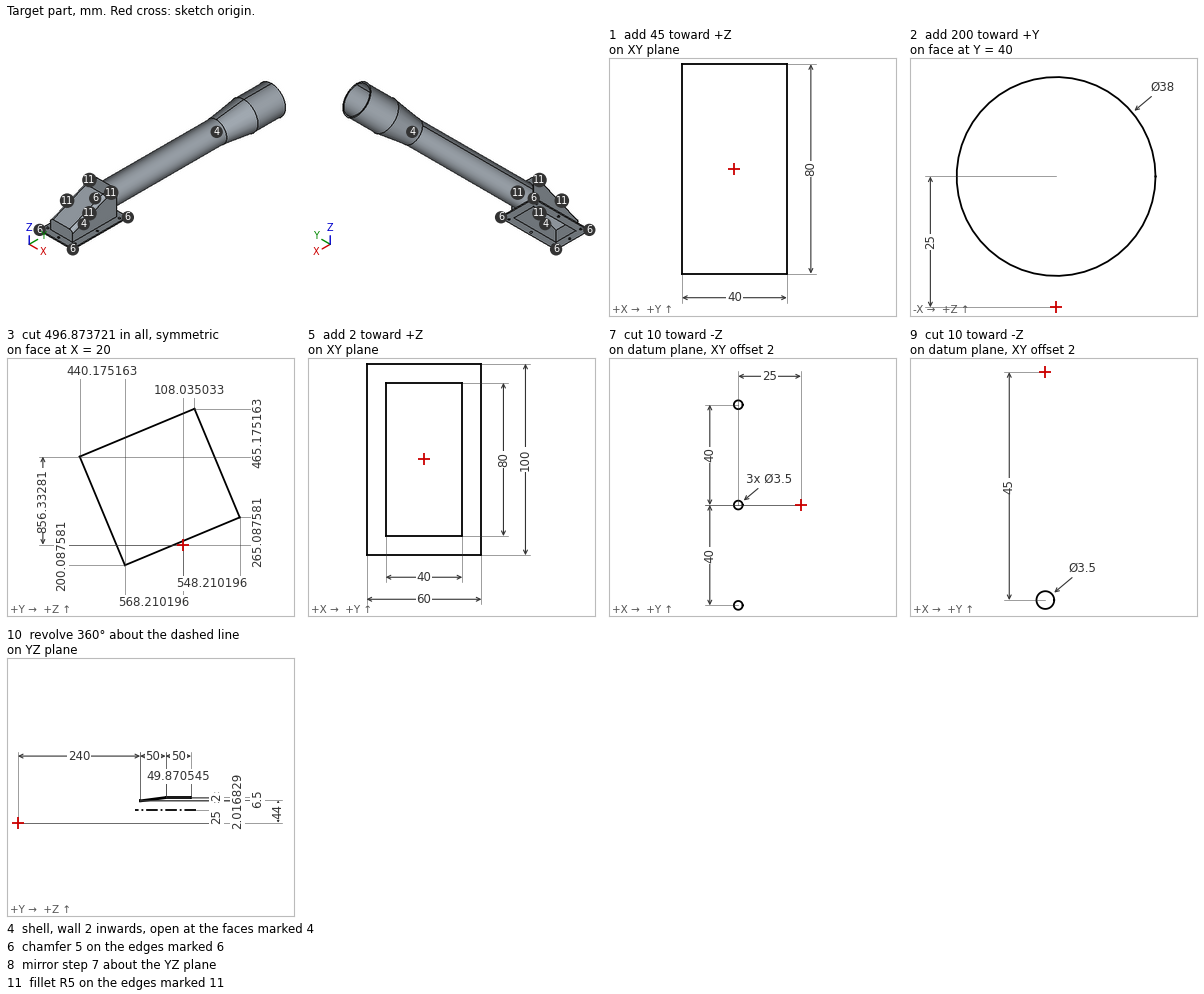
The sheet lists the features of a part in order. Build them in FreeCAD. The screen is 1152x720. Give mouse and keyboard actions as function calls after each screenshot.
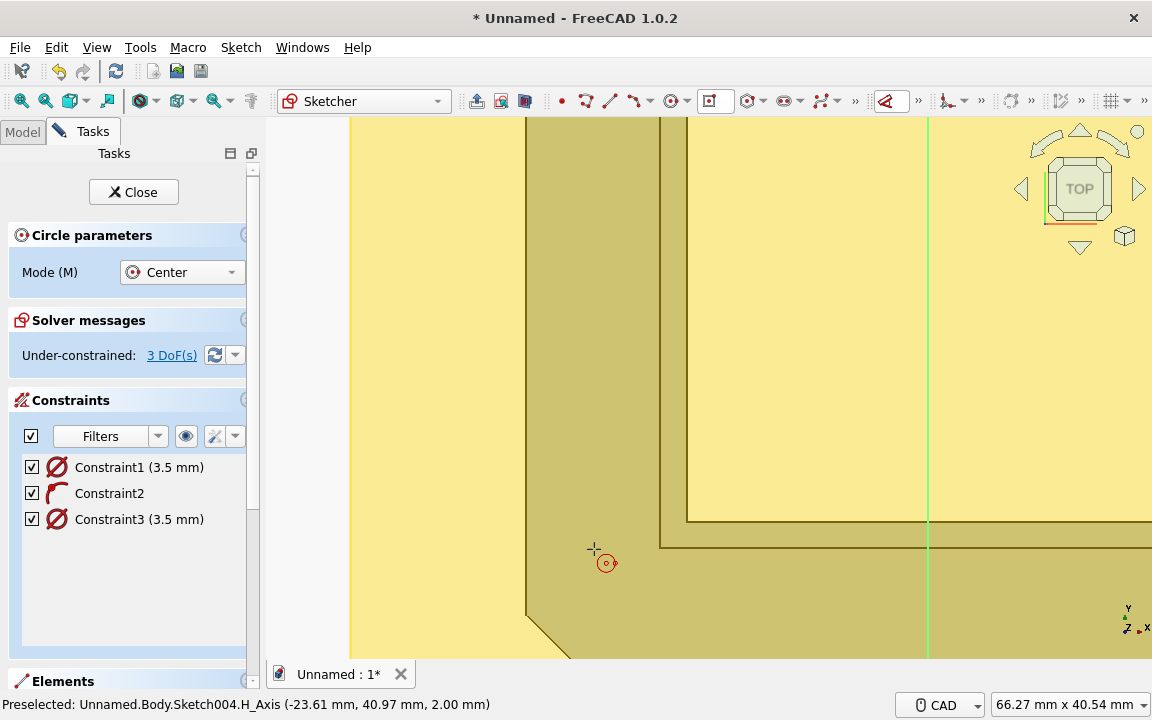
click(593, 548)
move(610, 532)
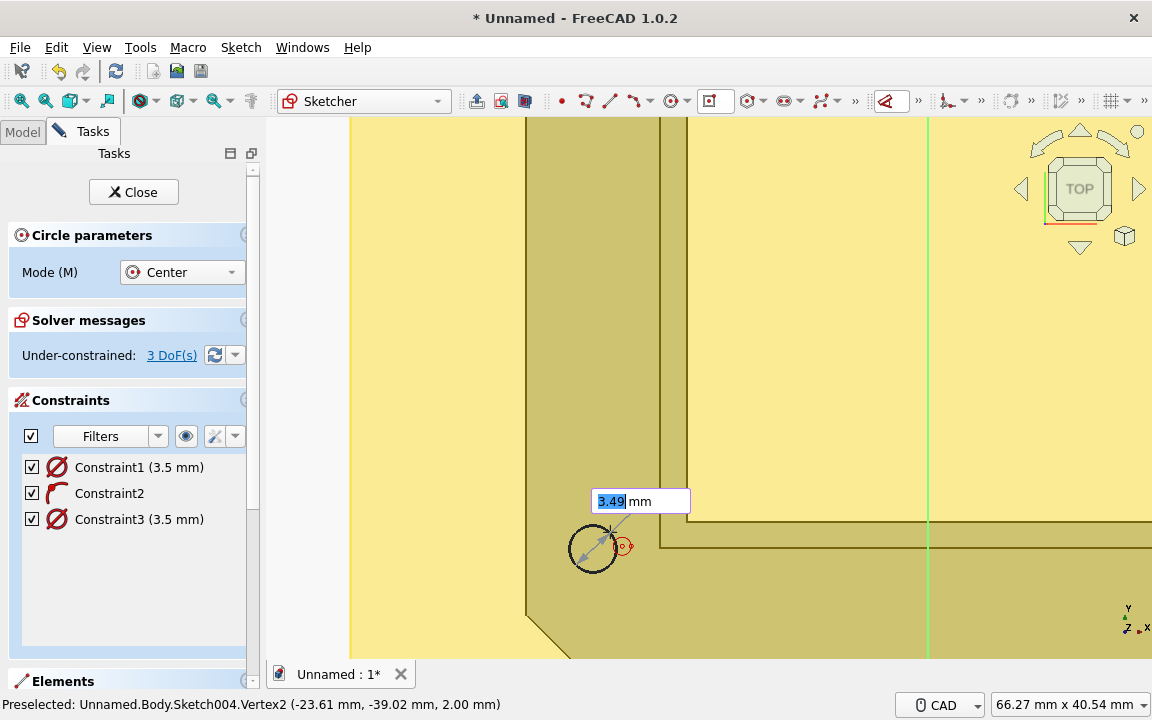
text(3.5)
key(Return)
key(Escape)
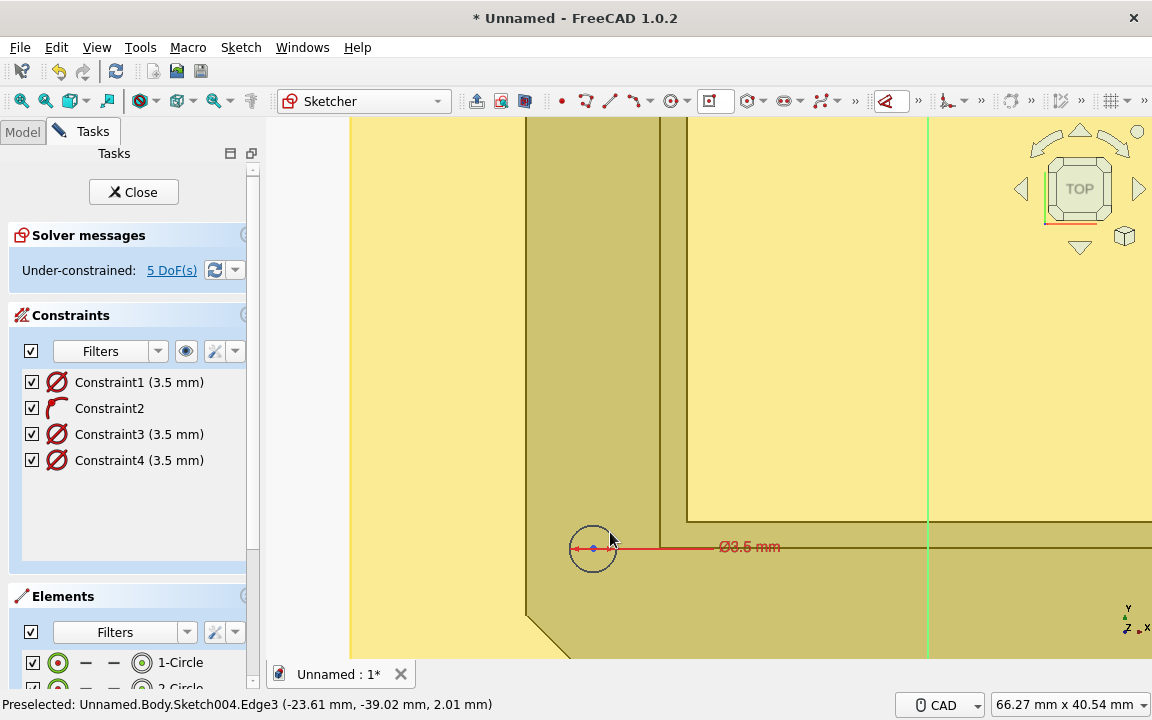
scroll(594, 549, down, 6)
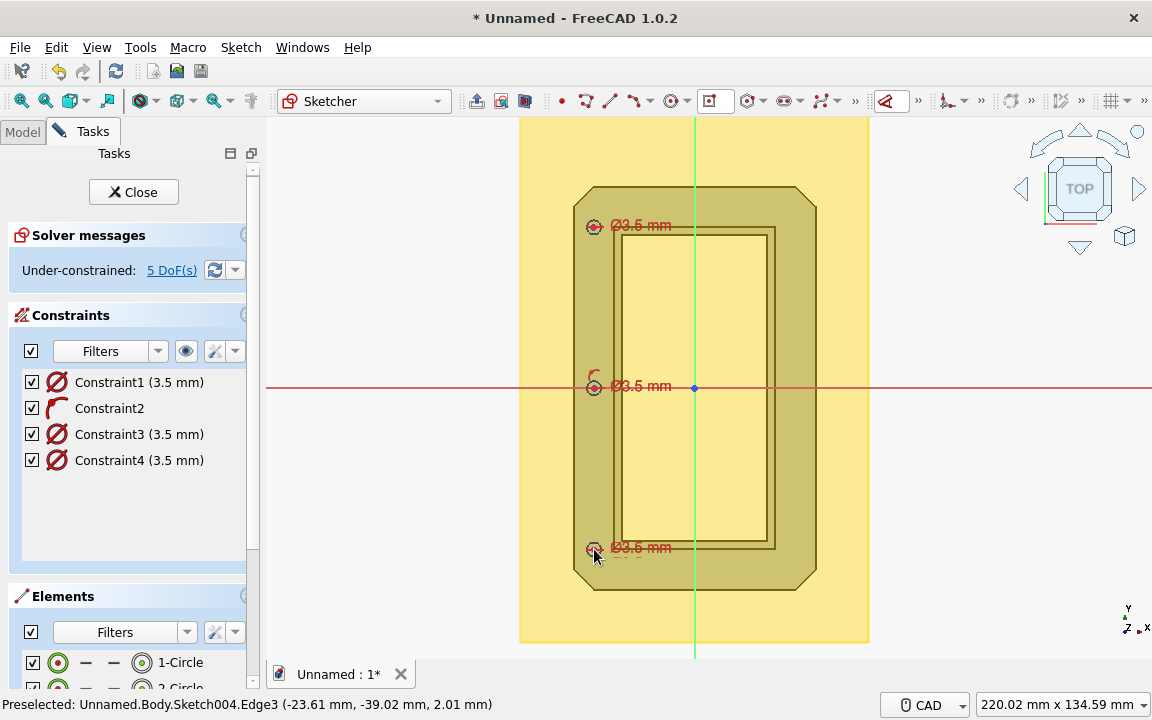
click(594, 388)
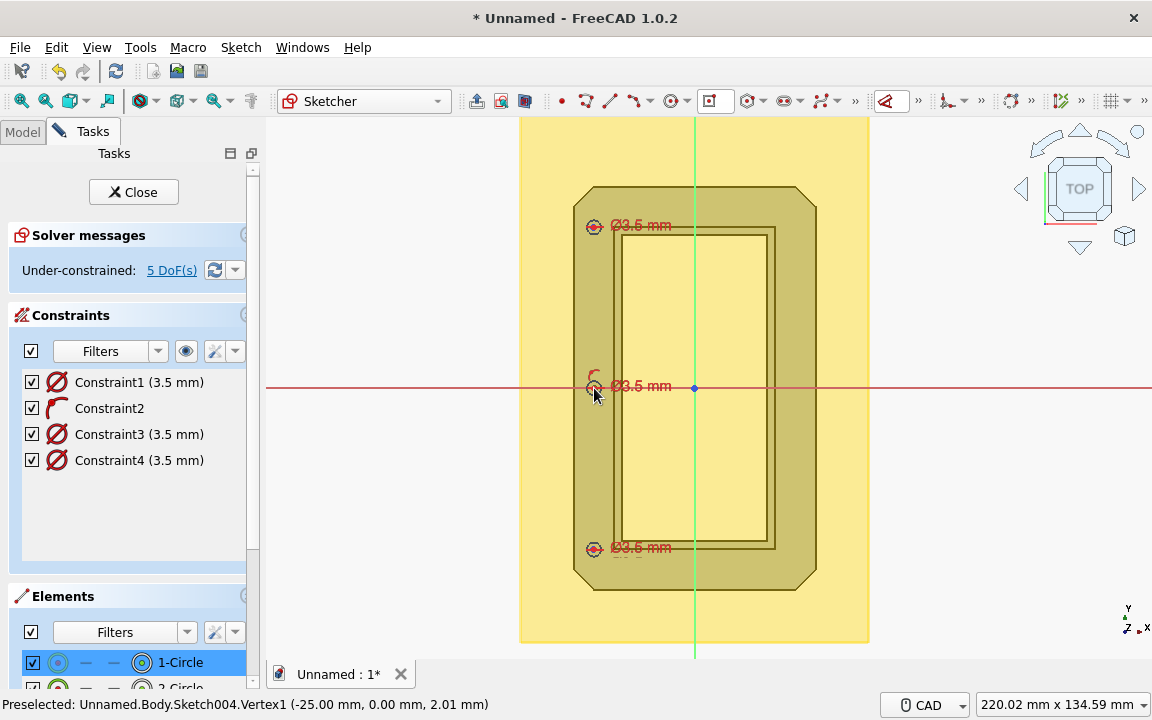
click(594, 227)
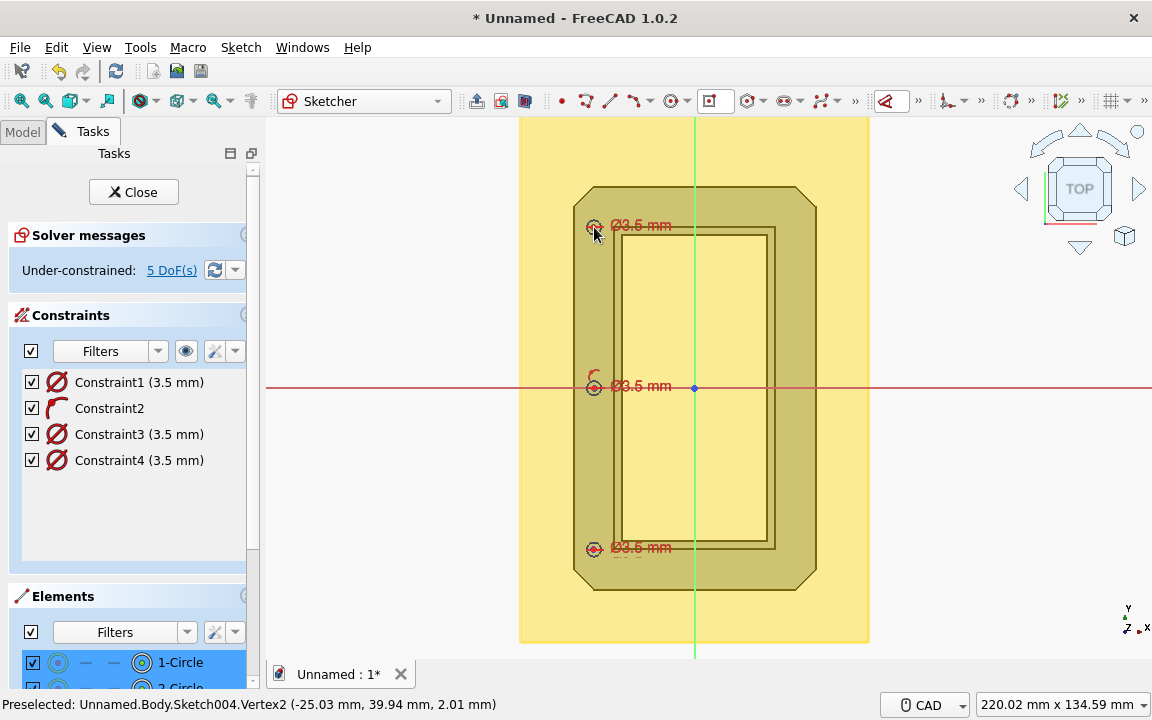
key(v)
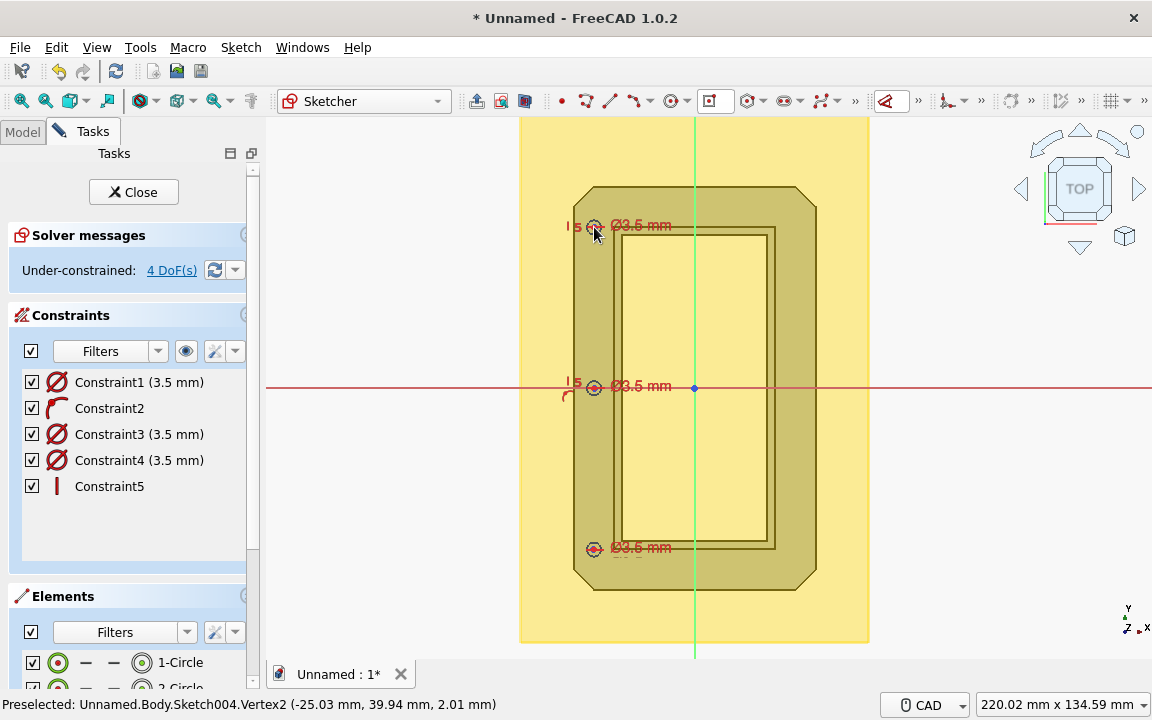
click(594, 388)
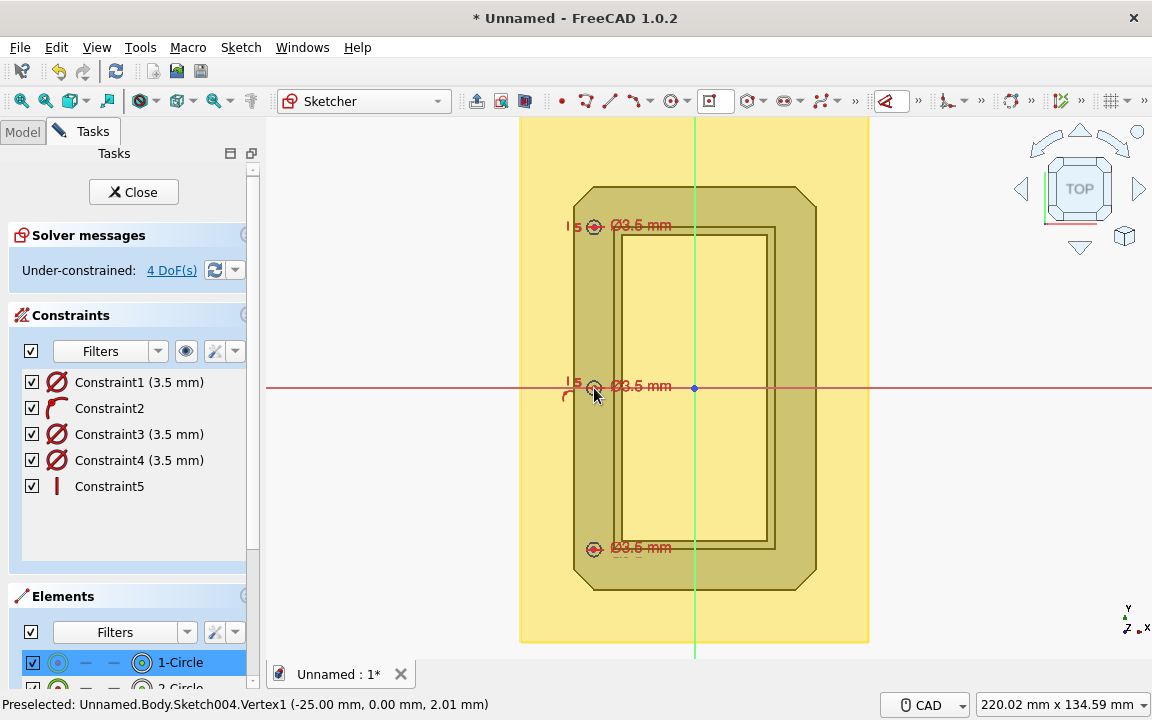
click(594, 550)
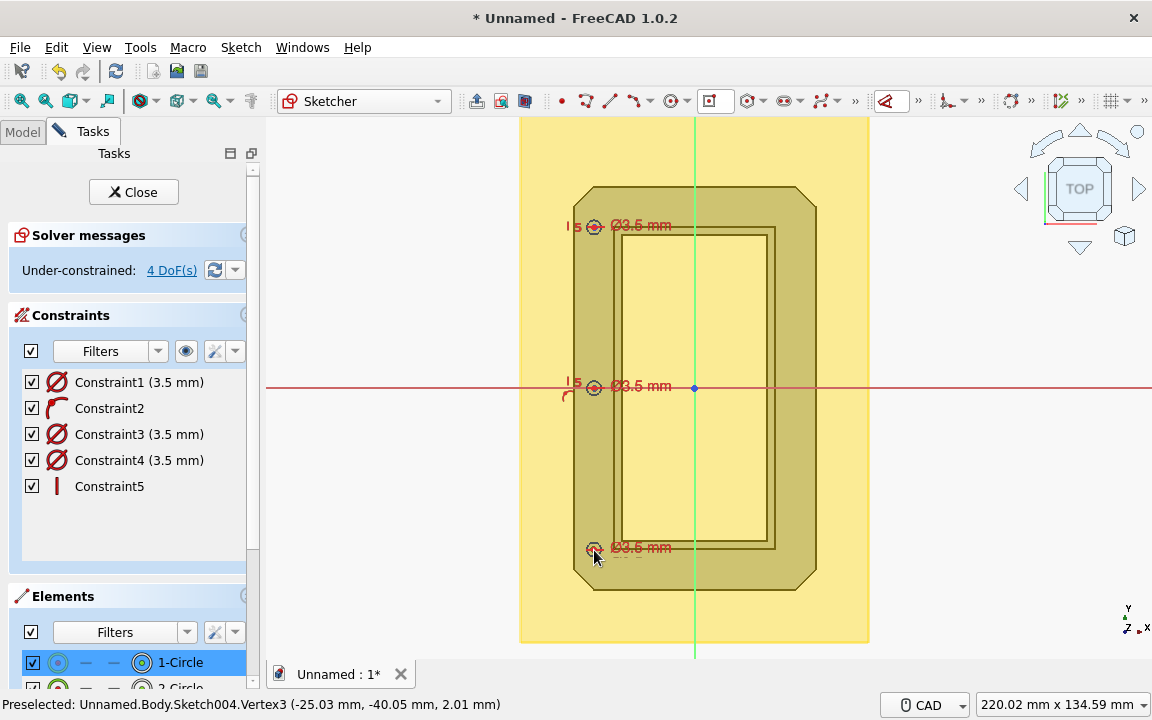
key(v)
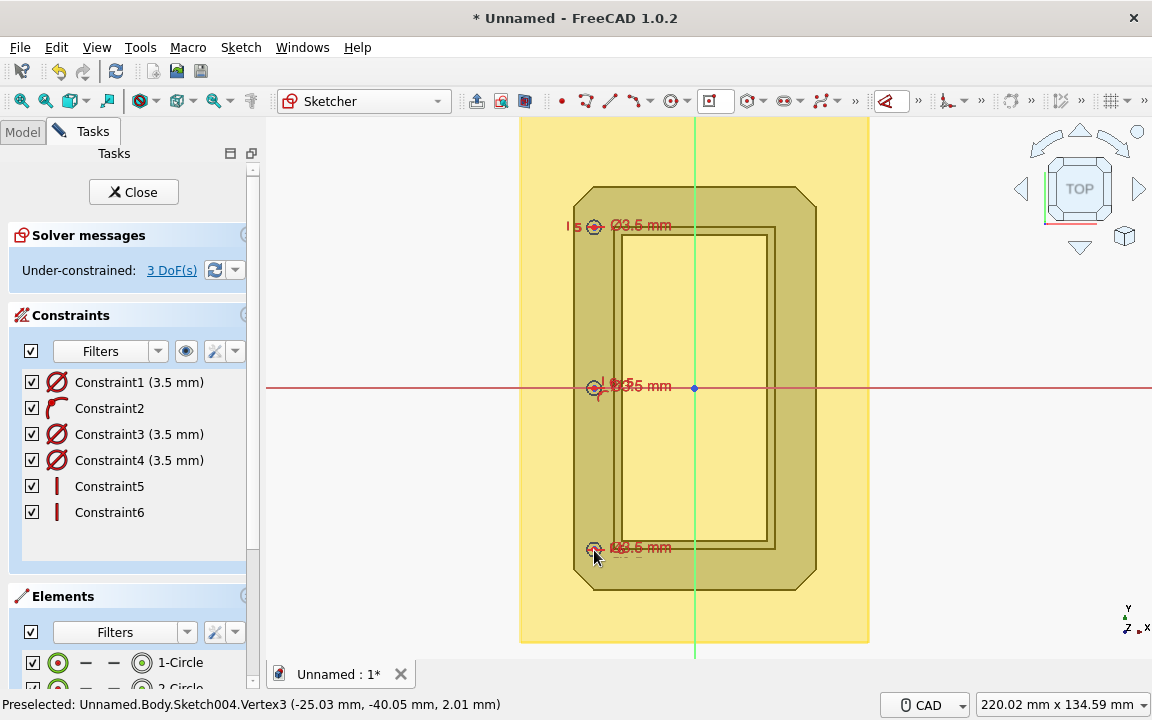
key(d)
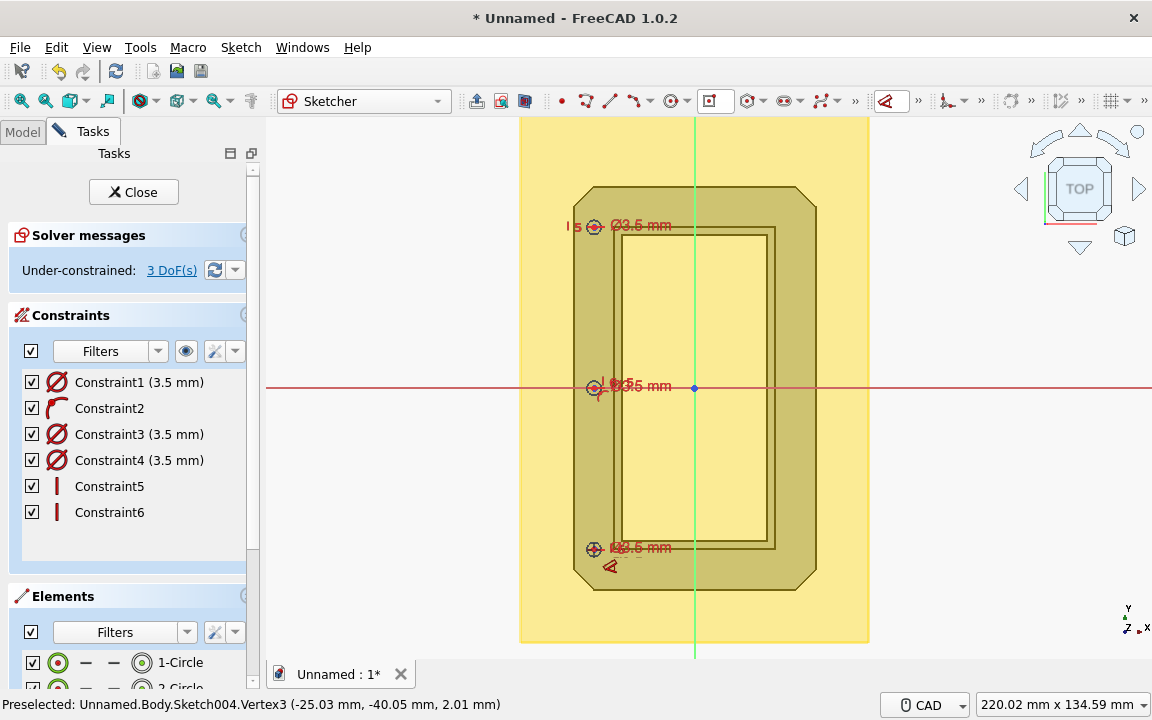
click(594, 388)
click(644, 422)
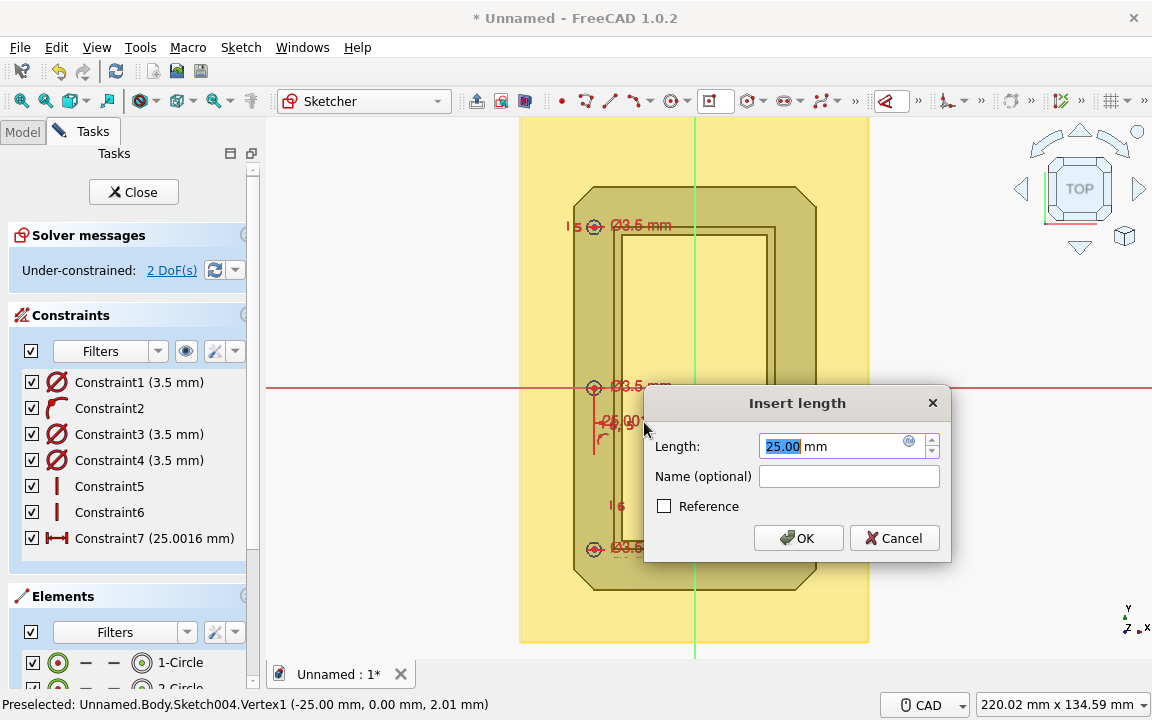
text(25)
key(Return)